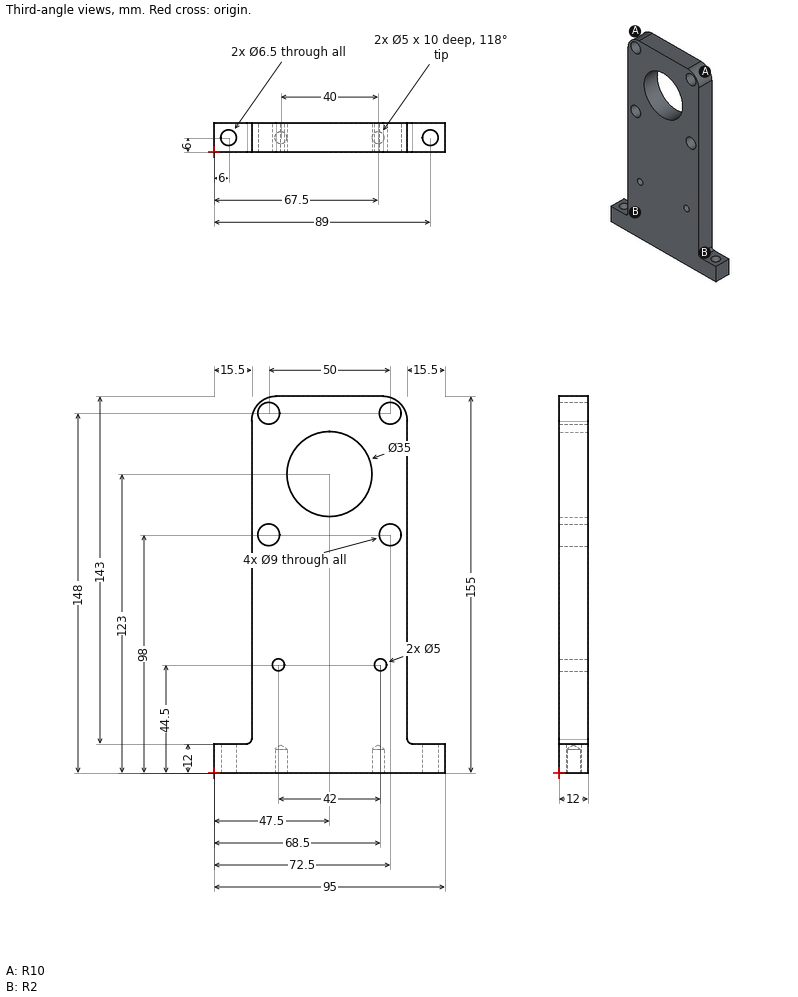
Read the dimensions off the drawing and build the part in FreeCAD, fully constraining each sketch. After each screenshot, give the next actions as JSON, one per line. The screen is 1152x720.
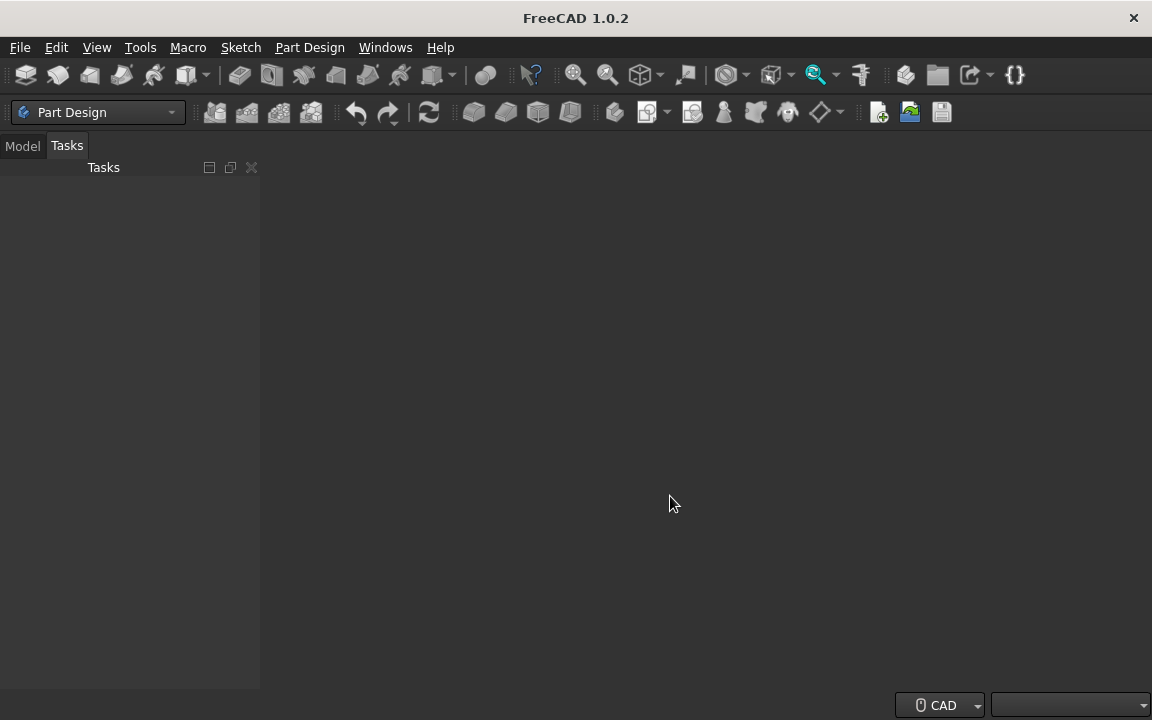
{"action": "left_click", "coordinate": [878, 112]}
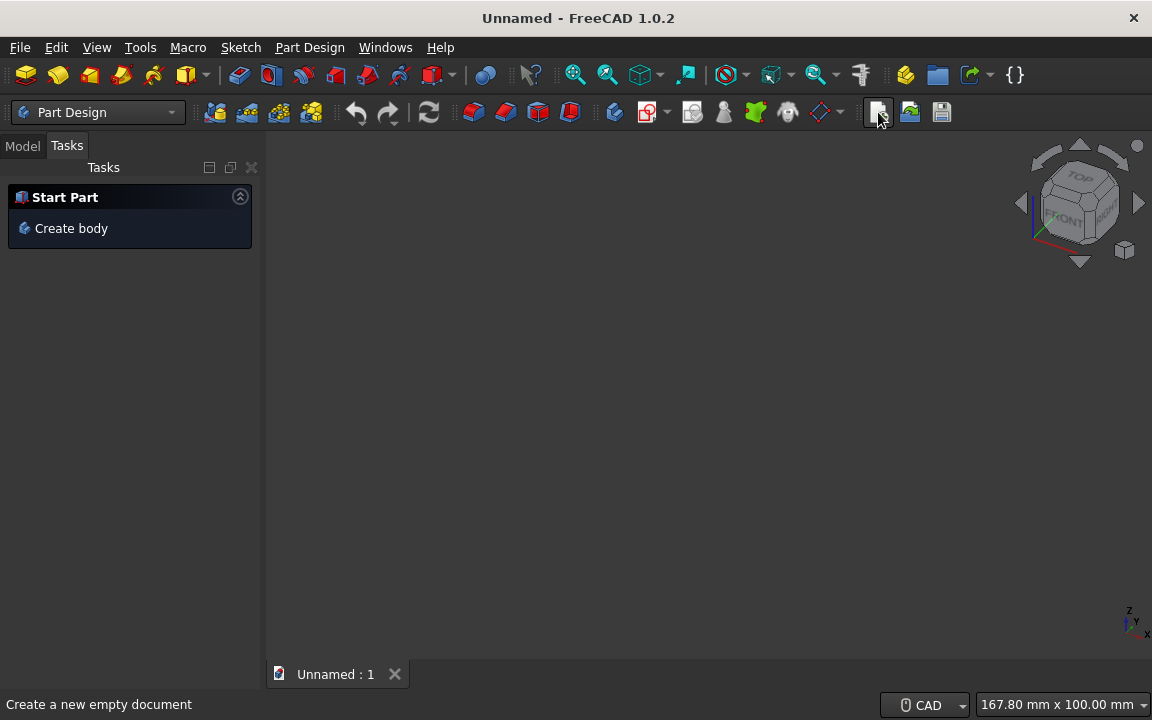
{"action": "left_click", "coordinate": [648, 112]}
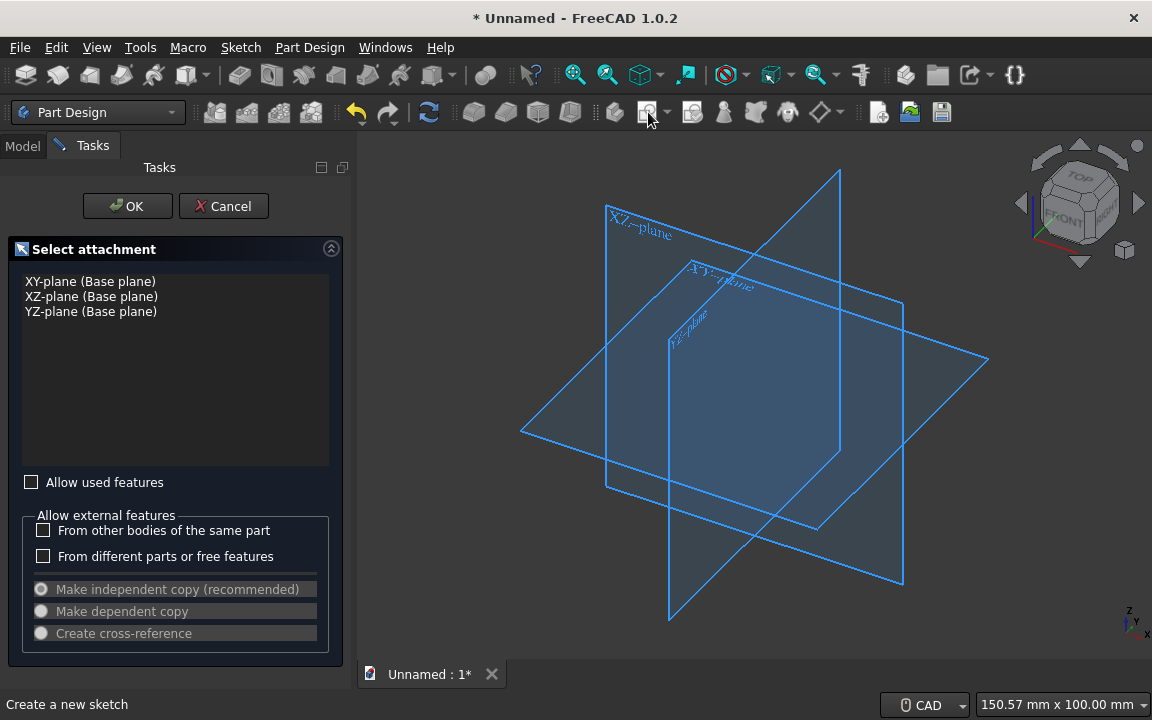
{"action": "left_click", "coordinate": [82, 296]}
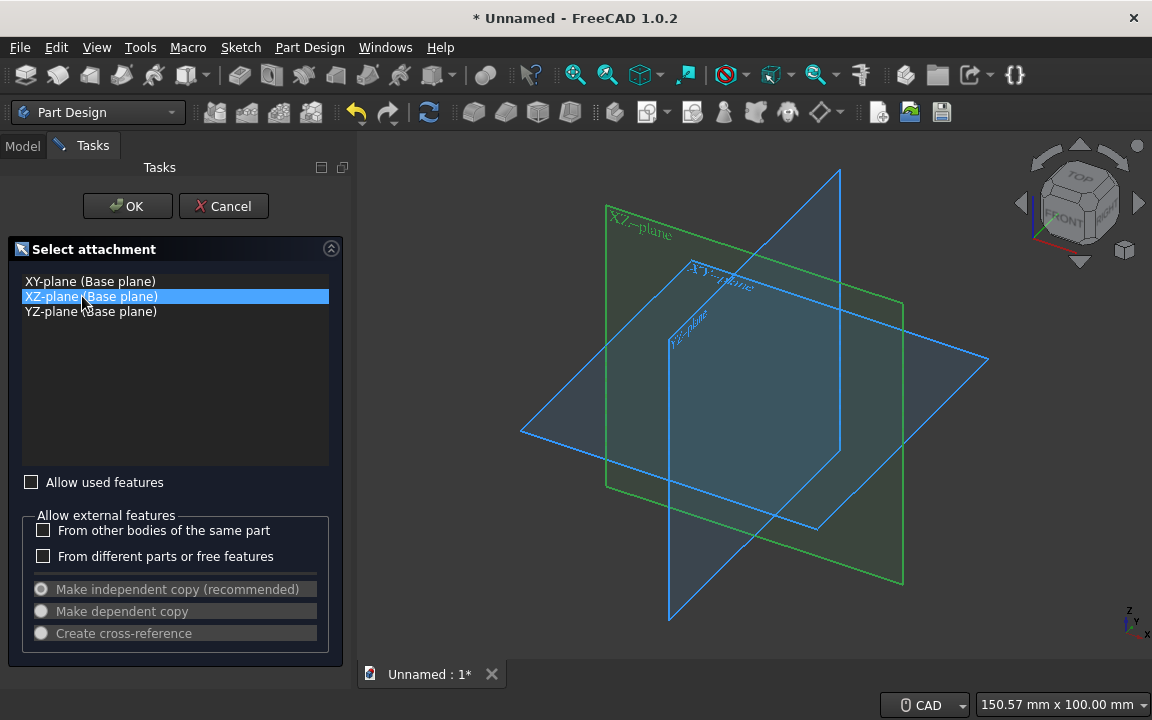
{"action": "left_click", "coordinate": [128, 206]}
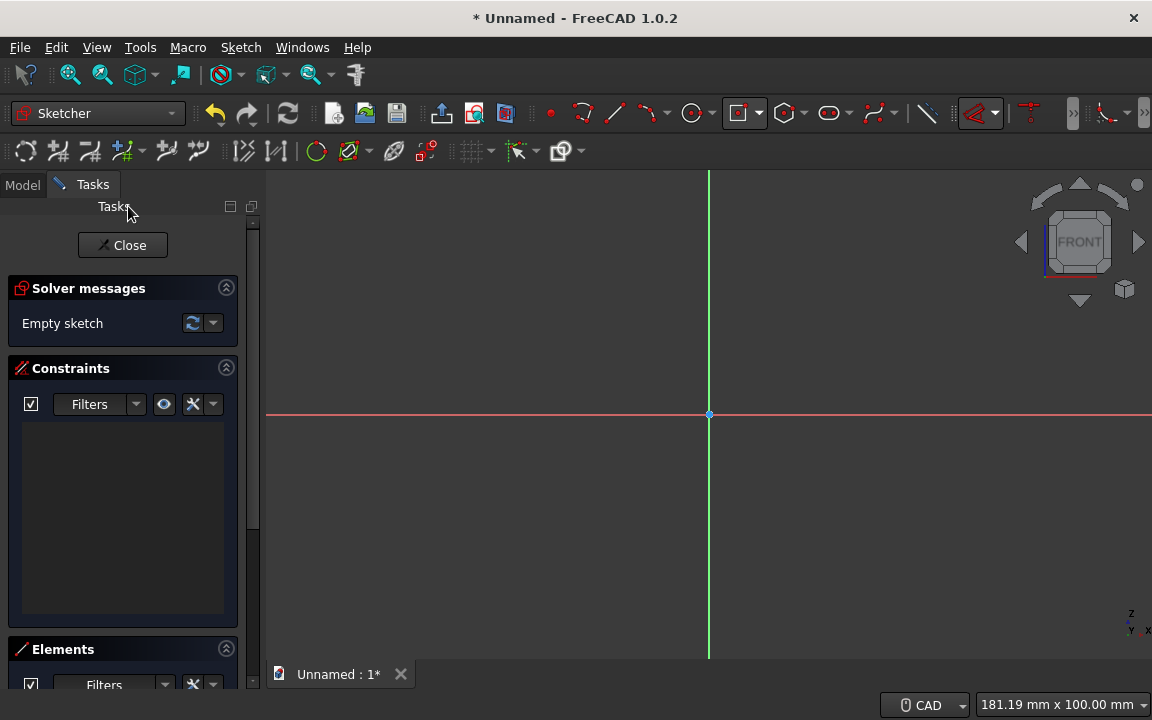
{"action": "scroll", "coordinate": [465, 631], "scroll_direction": "down", "scroll_amount": 5}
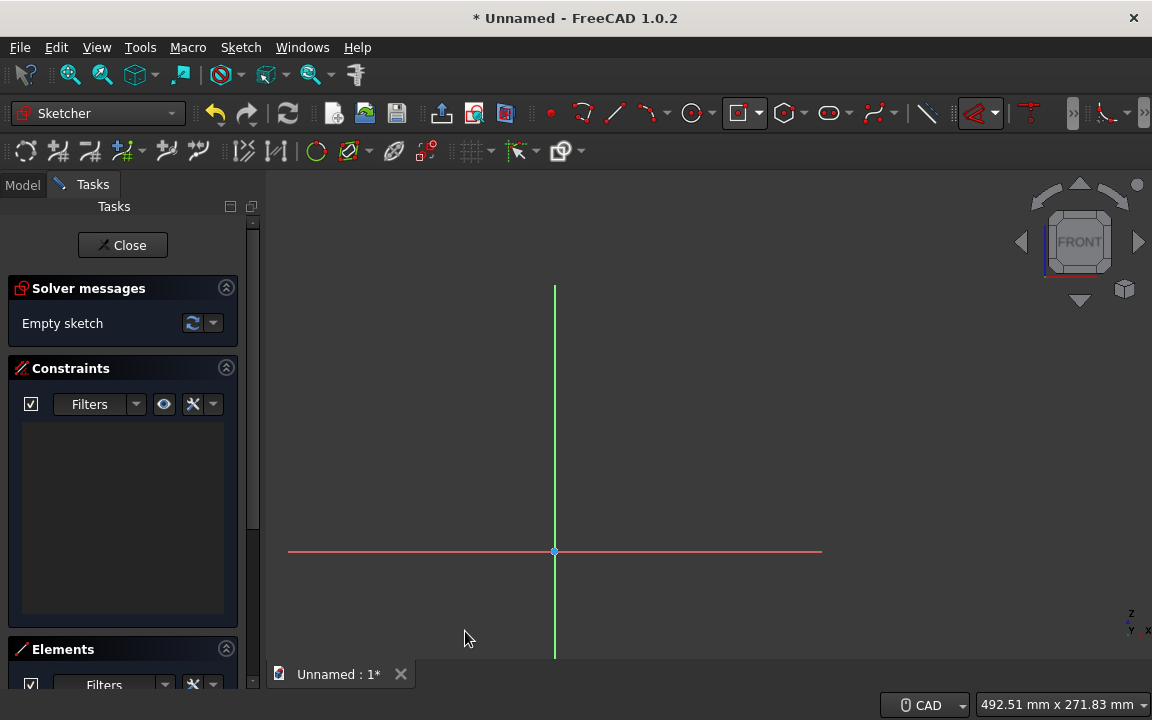
{"action": "key", "text": "g r"}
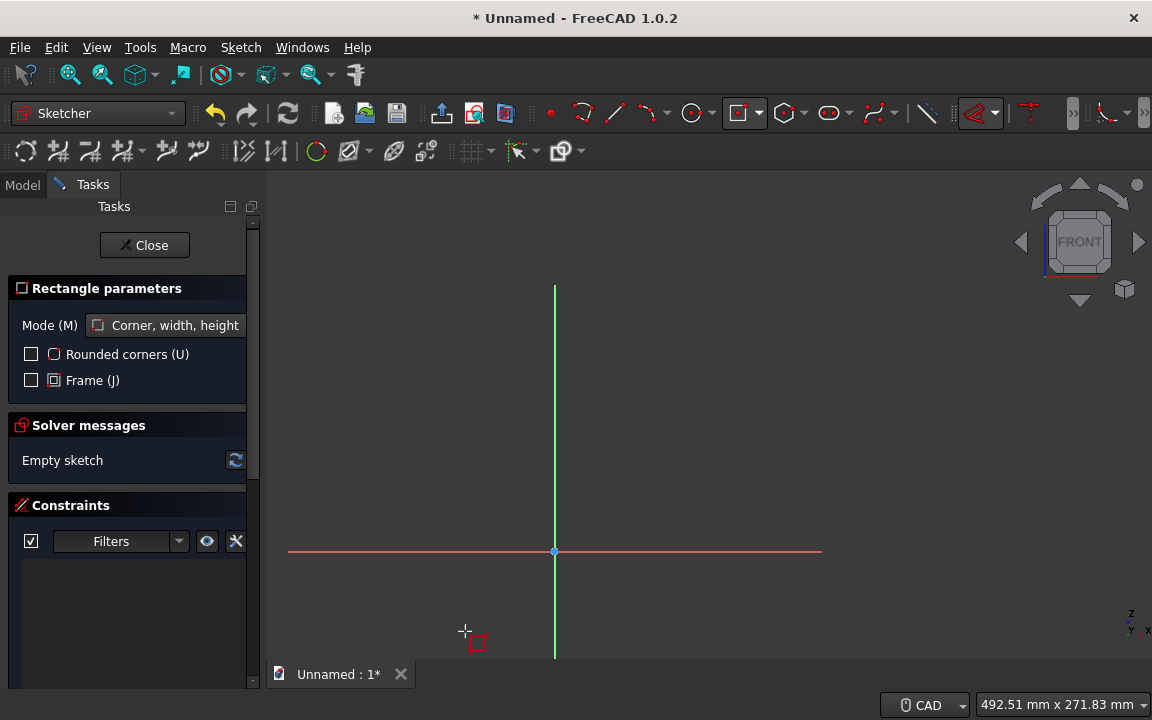
{"action": "left_click", "coordinate": [555, 552]}
{"action": "left_click", "coordinate": [726, 273]}
{"action": "key", "text": "Escape"}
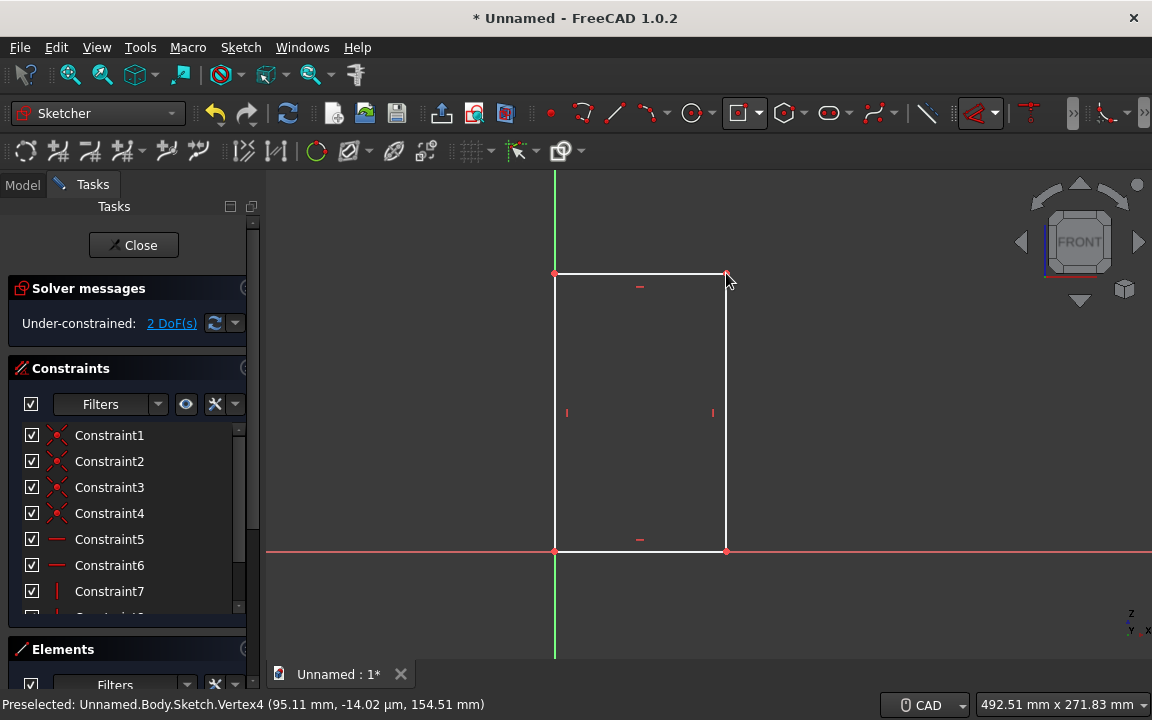
{"action": "left_click", "coordinate": [974, 114]}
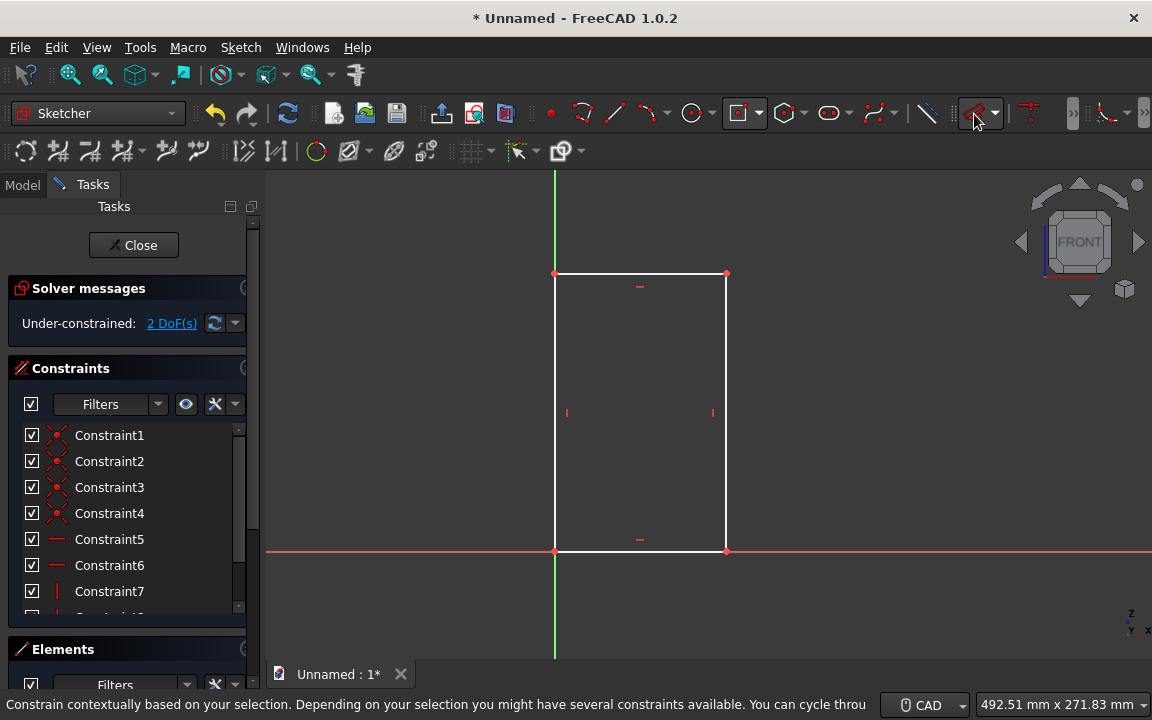
{"action": "left_click", "coordinate": [606, 552]}
{"action": "left_click", "coordinate": [640, 586]}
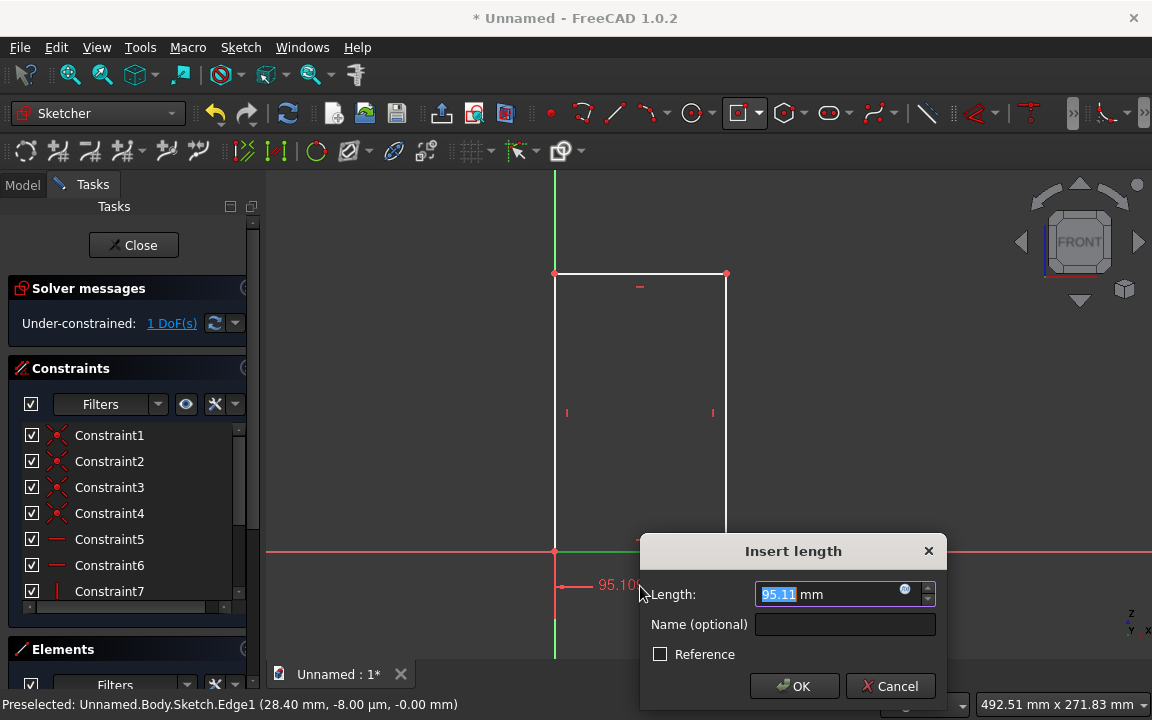
{"action": "type", "text": "95"}
{"action": "key", "text": "Return"}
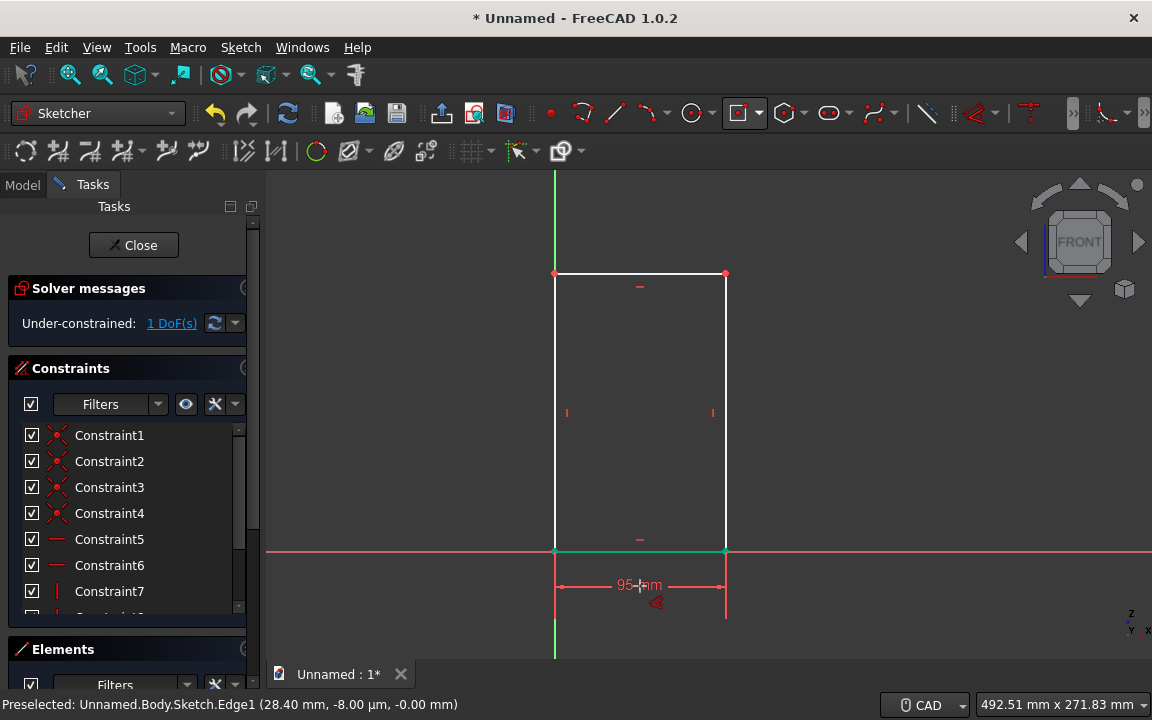
{"action": "left_click", "coordinate": [726, 469]}
{"action": "left_click", "coordinate": [760, 413]}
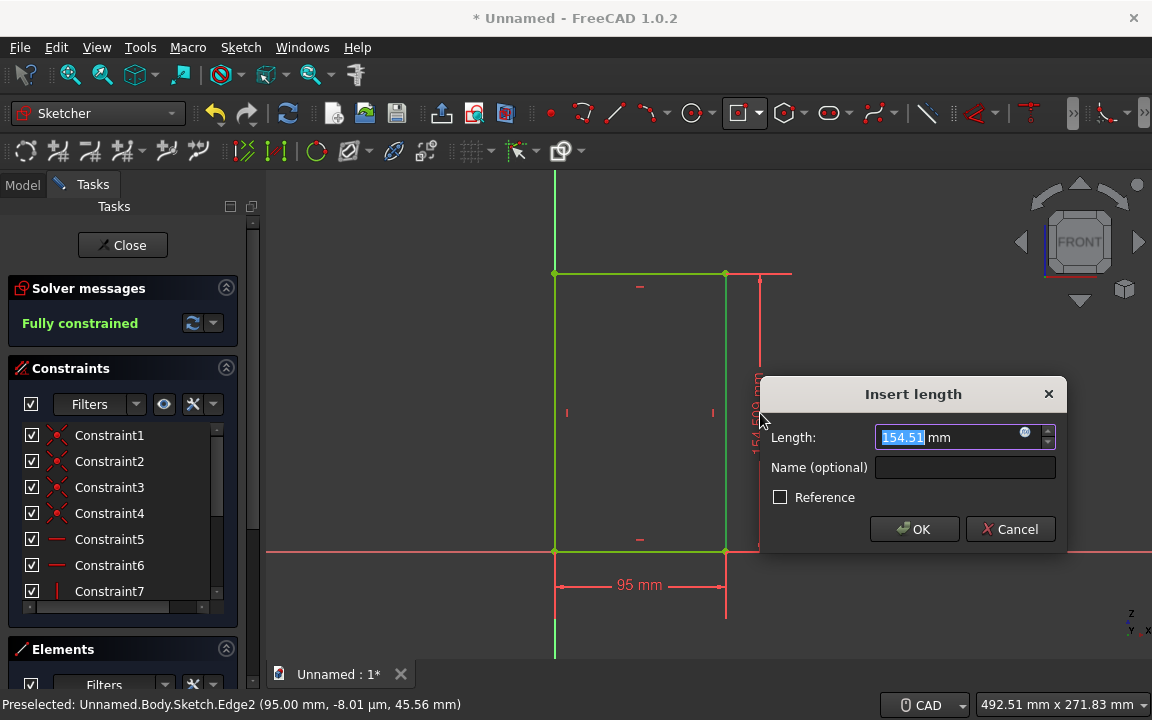
{"action": "type", "text": "155"}
{"action": "key", "text": "Return"}
{"action": "key", "text": "Escape"}